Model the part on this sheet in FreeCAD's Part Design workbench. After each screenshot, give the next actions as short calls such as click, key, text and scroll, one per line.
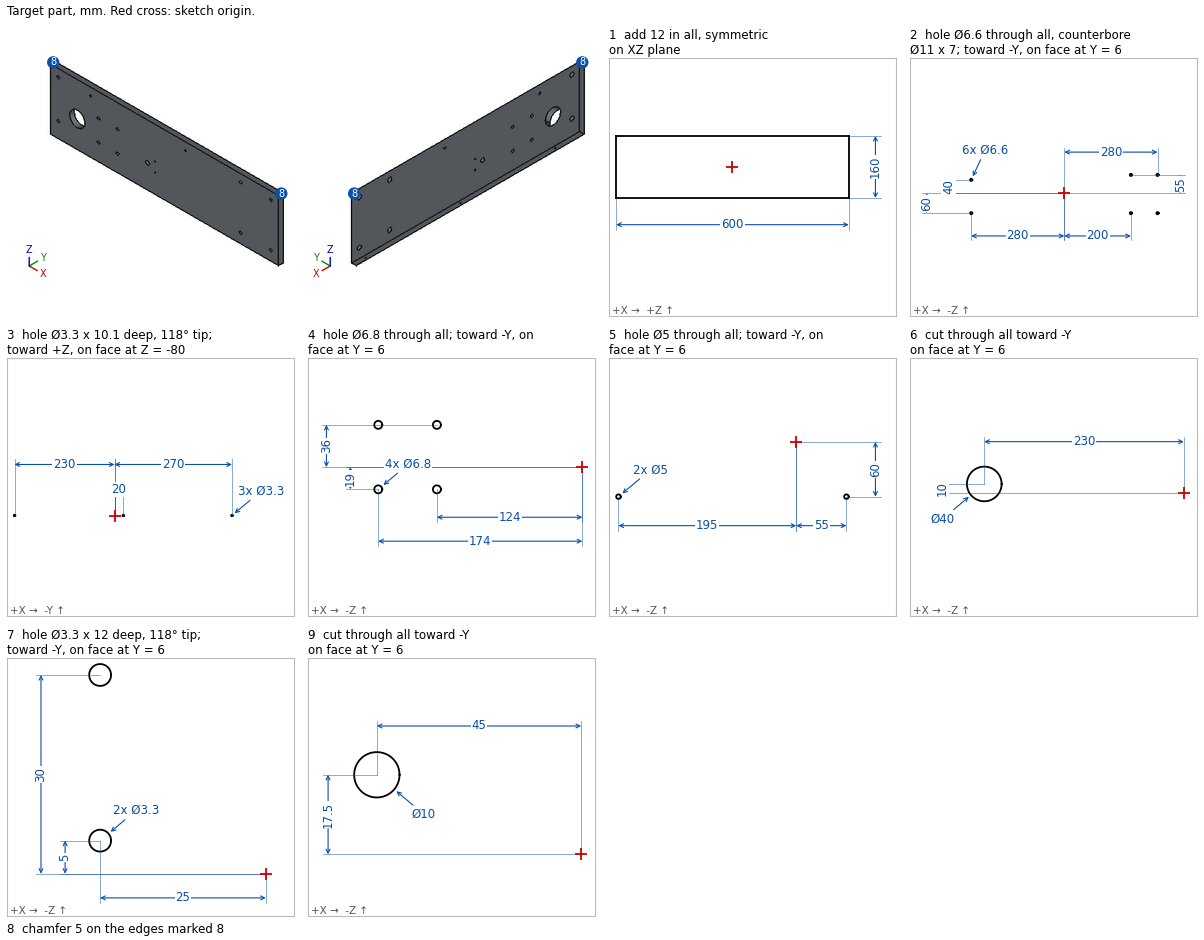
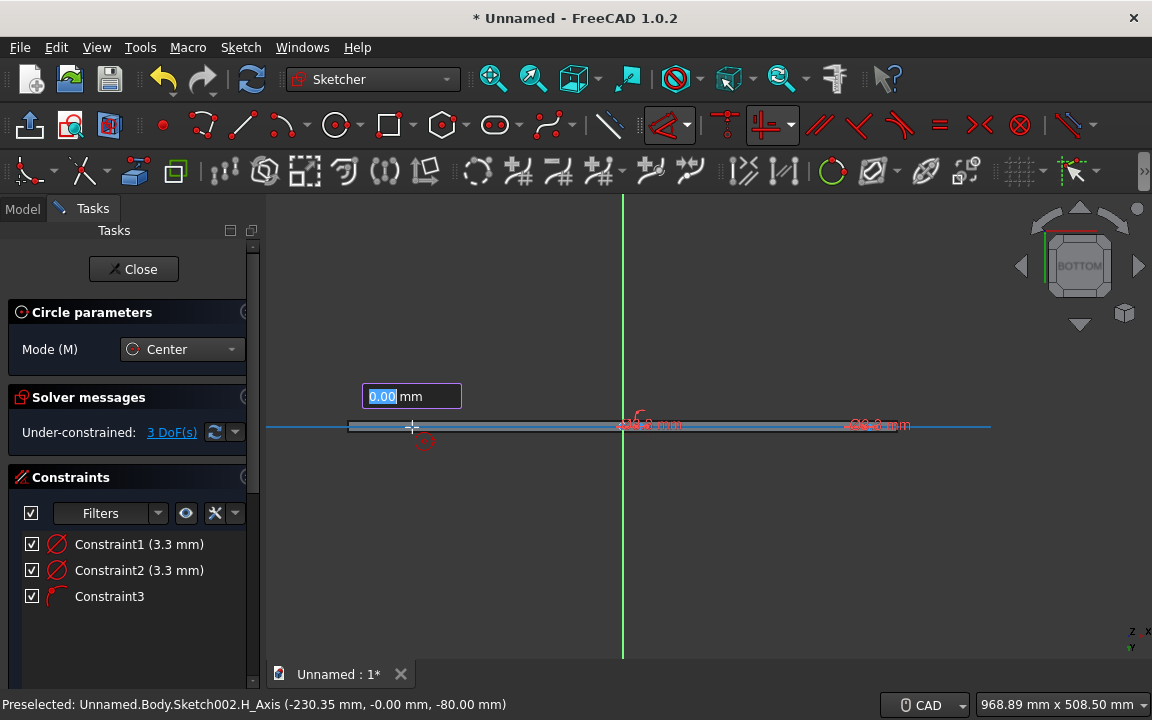
scroll(412, 428, up, 13)
move(407, 421)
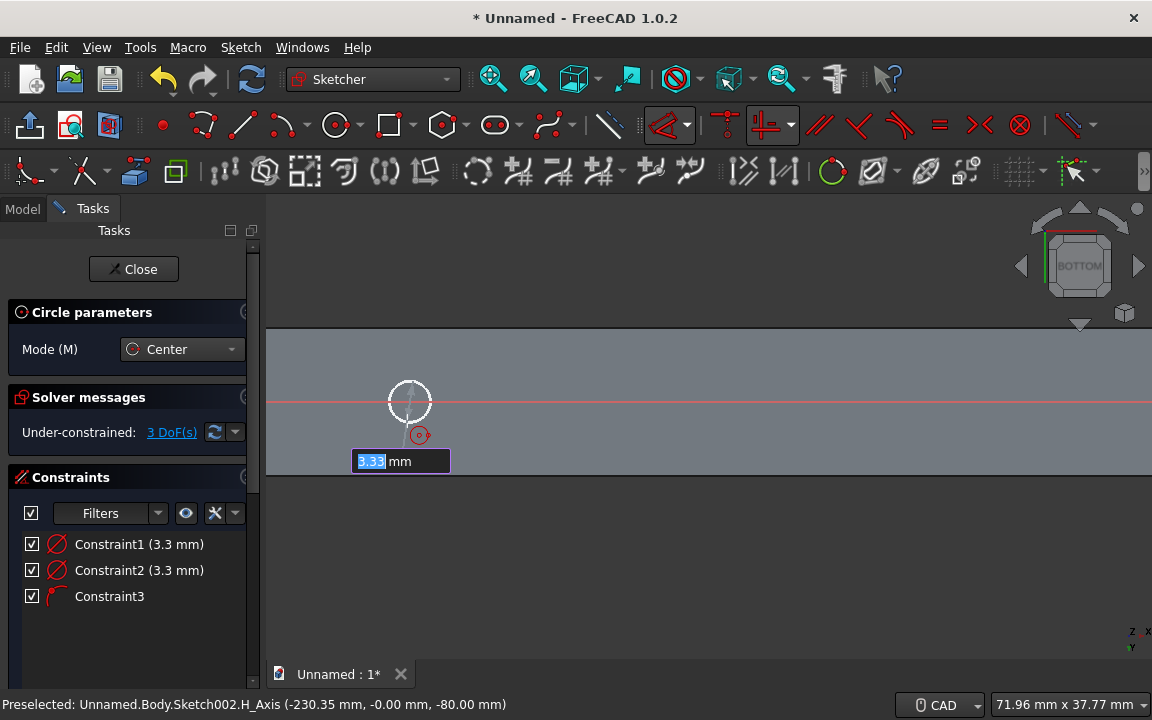
text(3.3)
key(Return)
key(Escape)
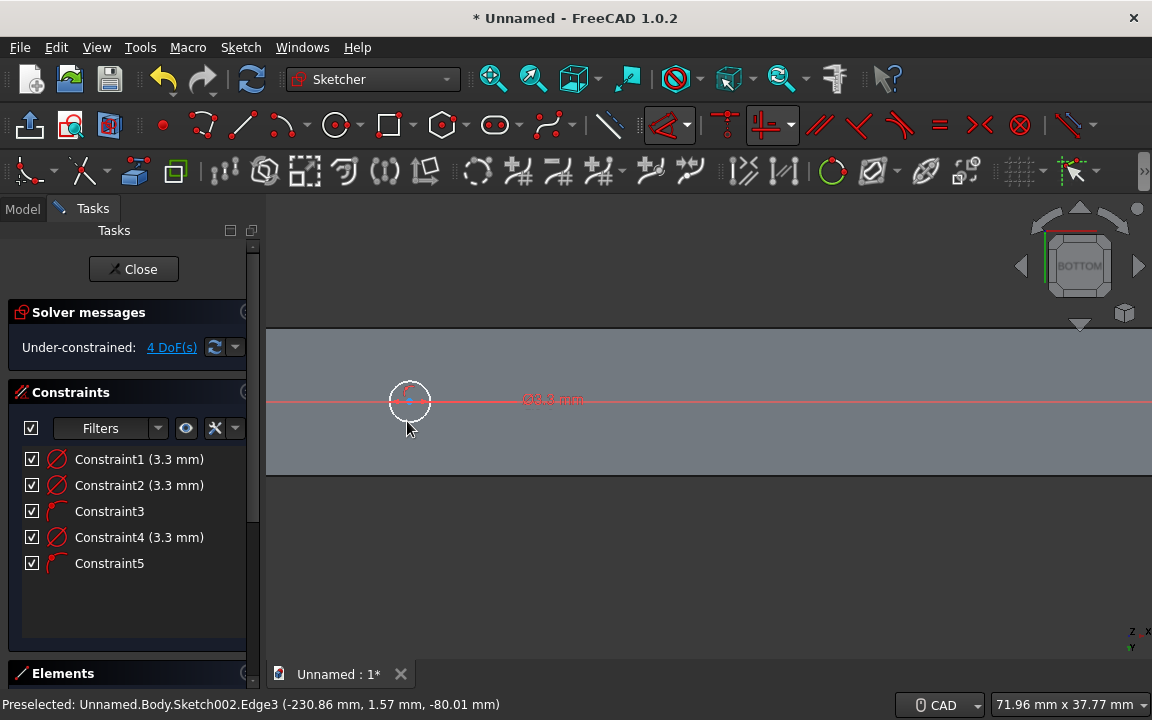
scroll(412, 428, down, 13)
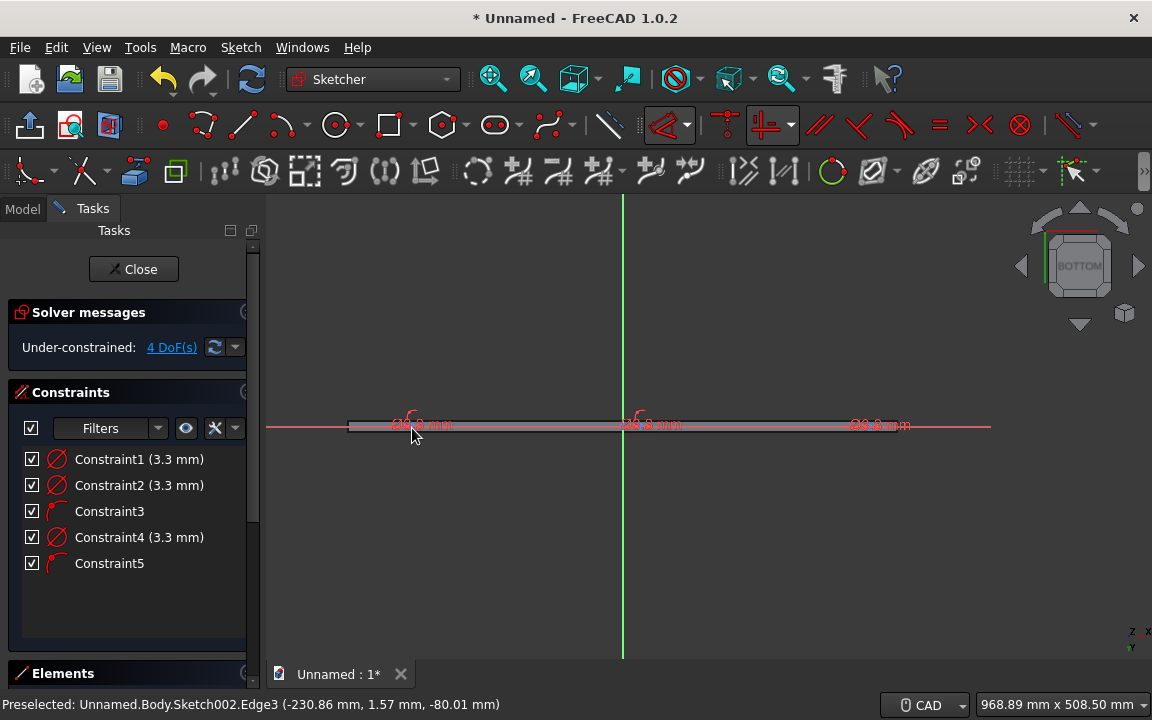
click(870, 427)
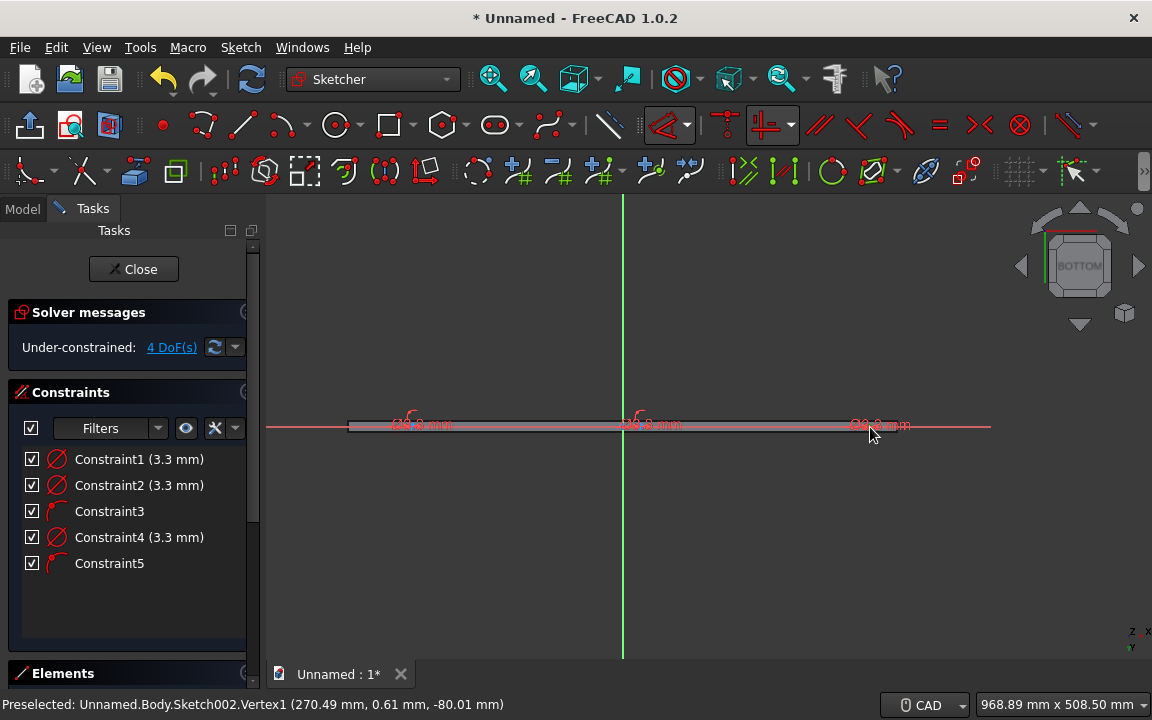
click(343, 427)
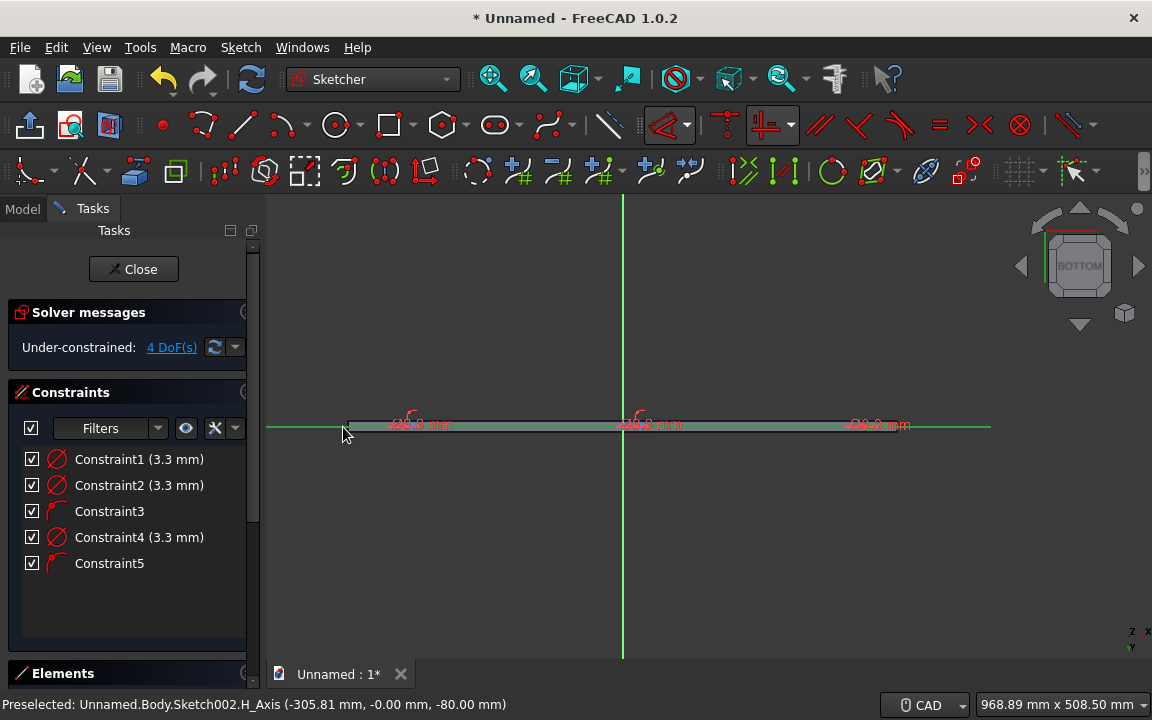
click(726, 126)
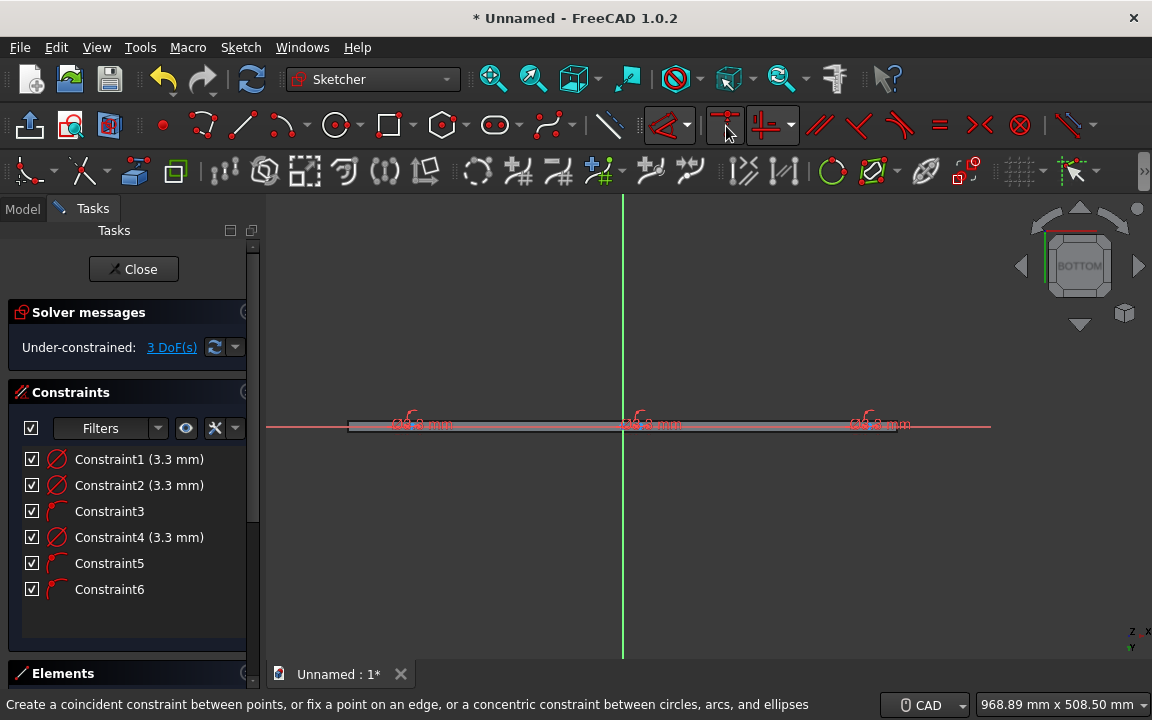
scroll(641, 427, up, 4)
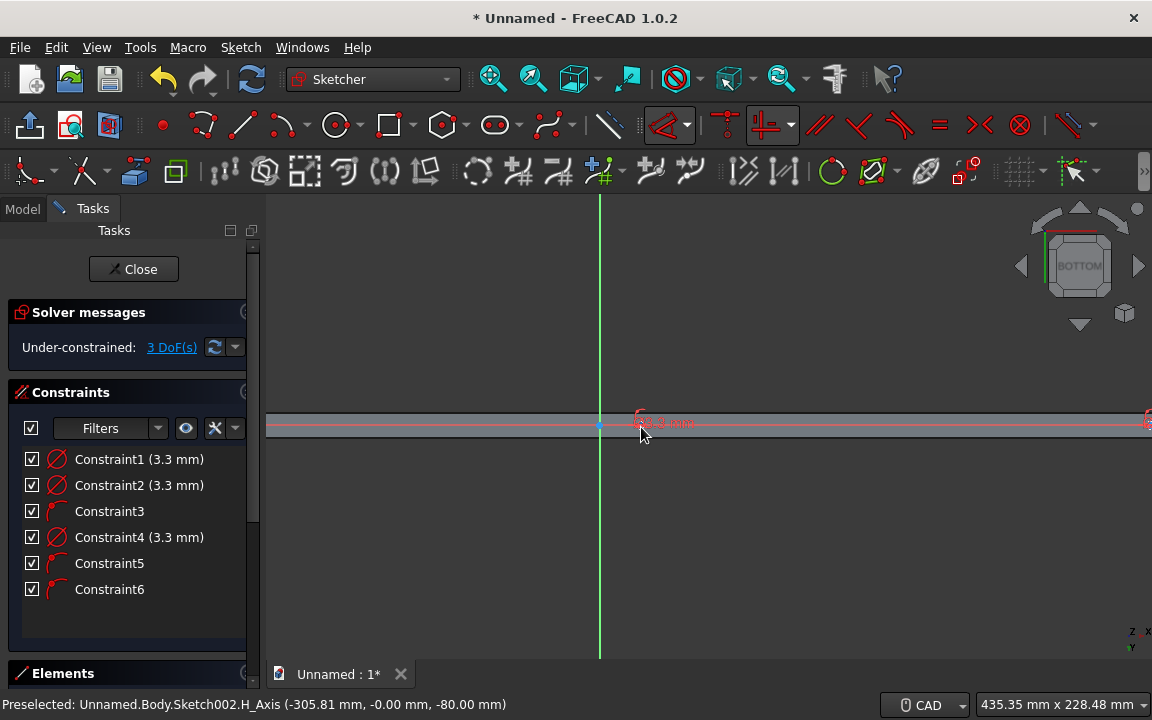
click(640, 425)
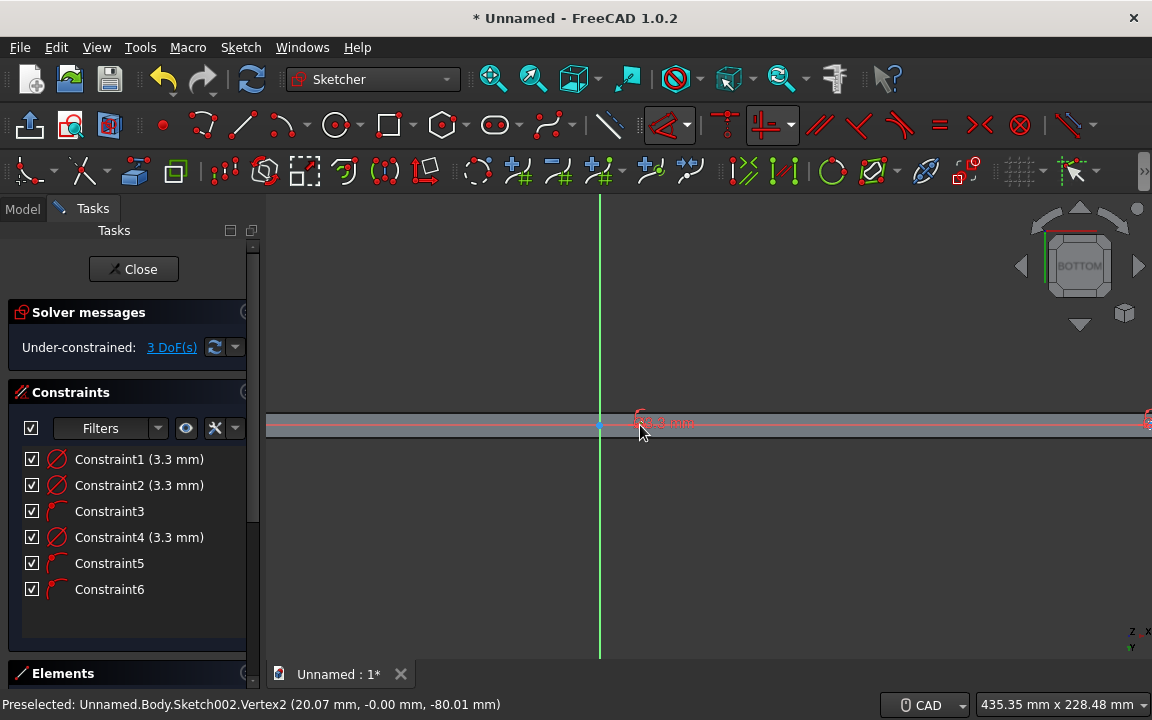
key(l)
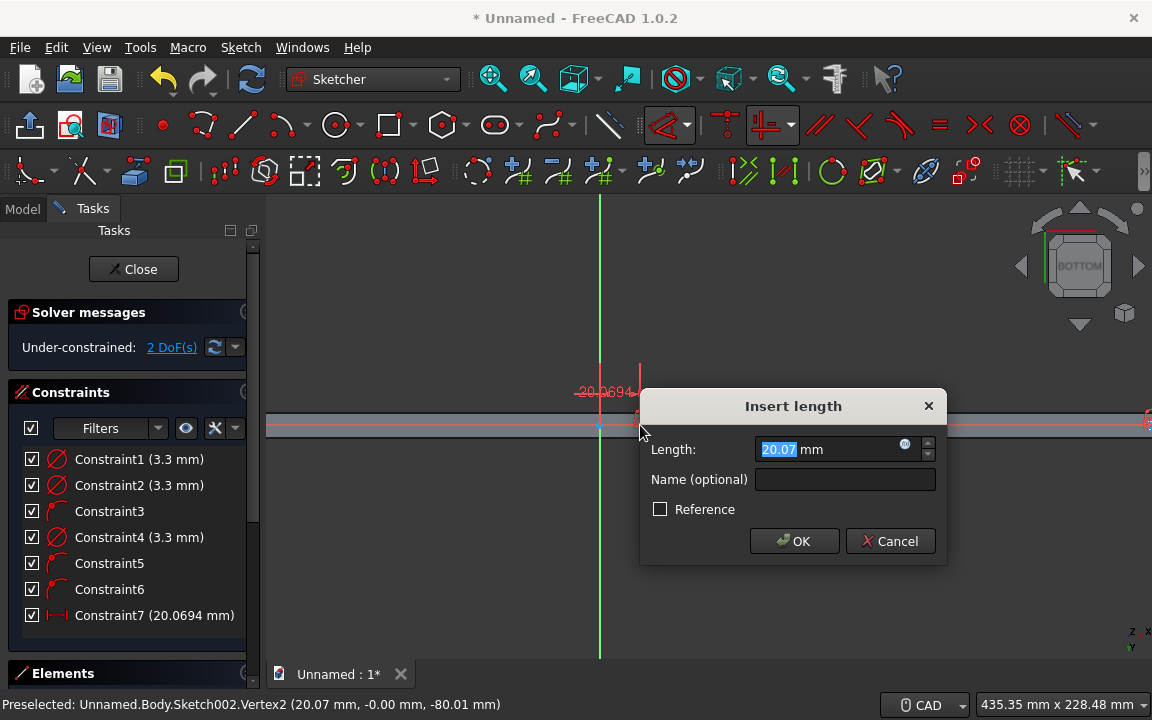
text(20)
key(Return)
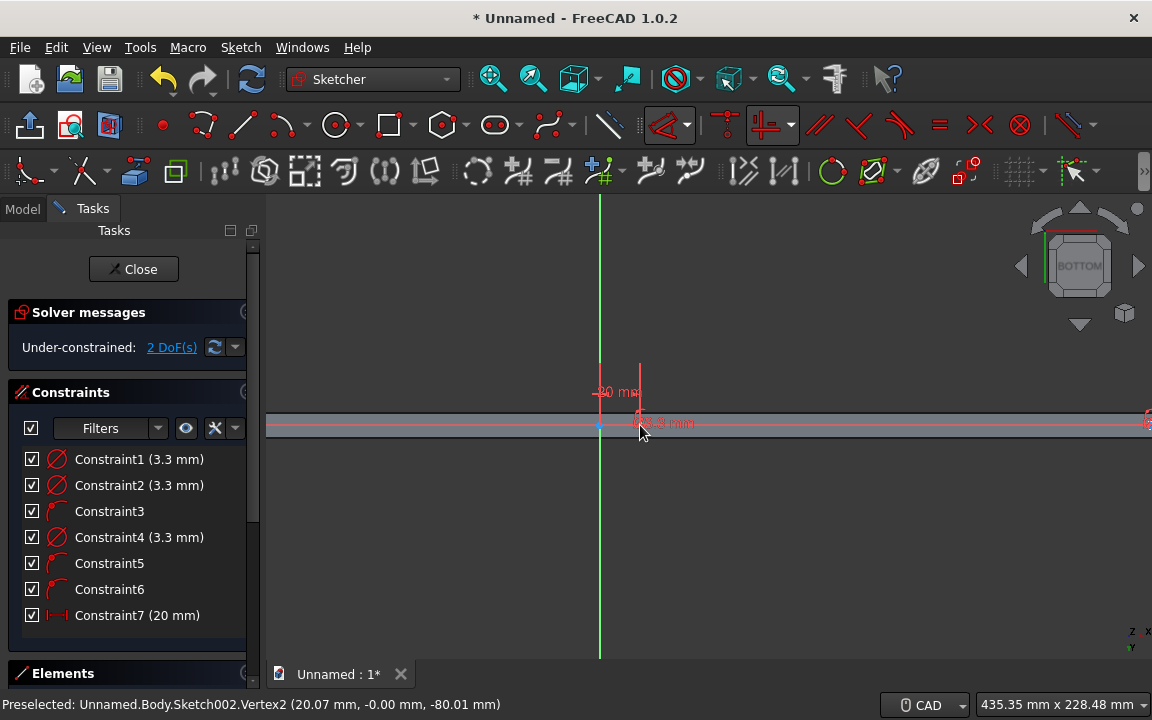
scroll(641, 427, down, 4)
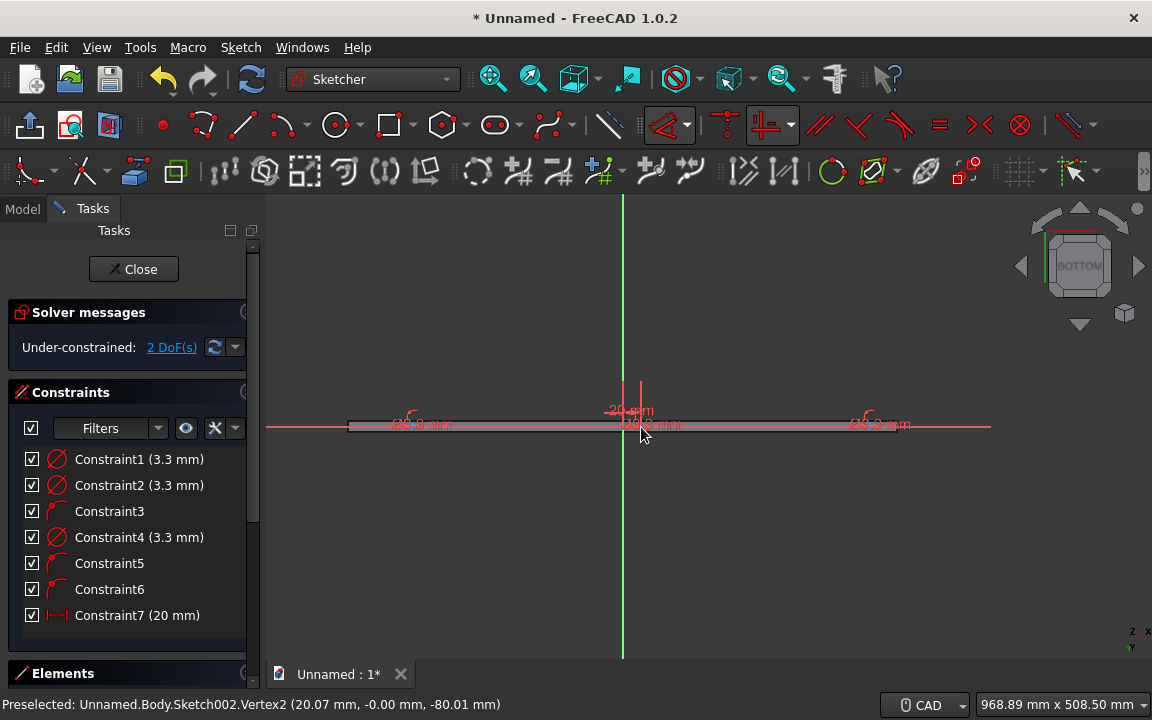
click(870, 427)